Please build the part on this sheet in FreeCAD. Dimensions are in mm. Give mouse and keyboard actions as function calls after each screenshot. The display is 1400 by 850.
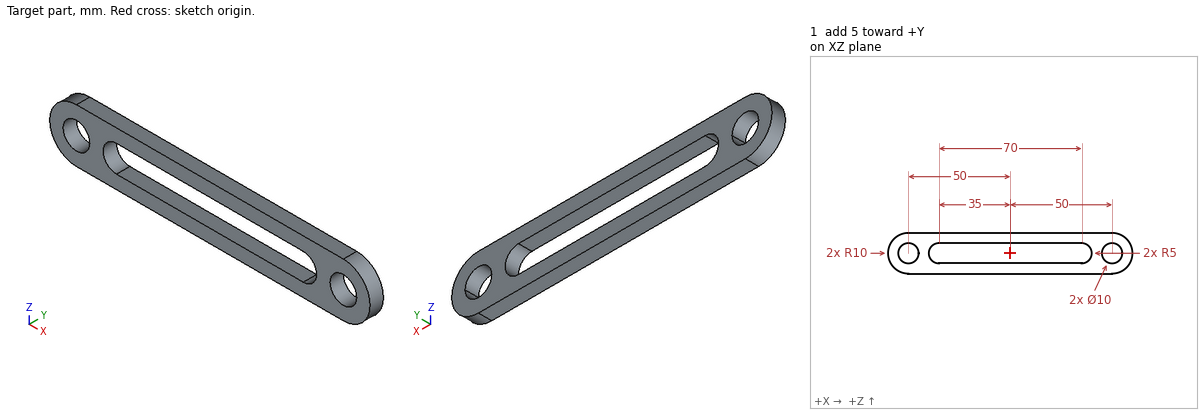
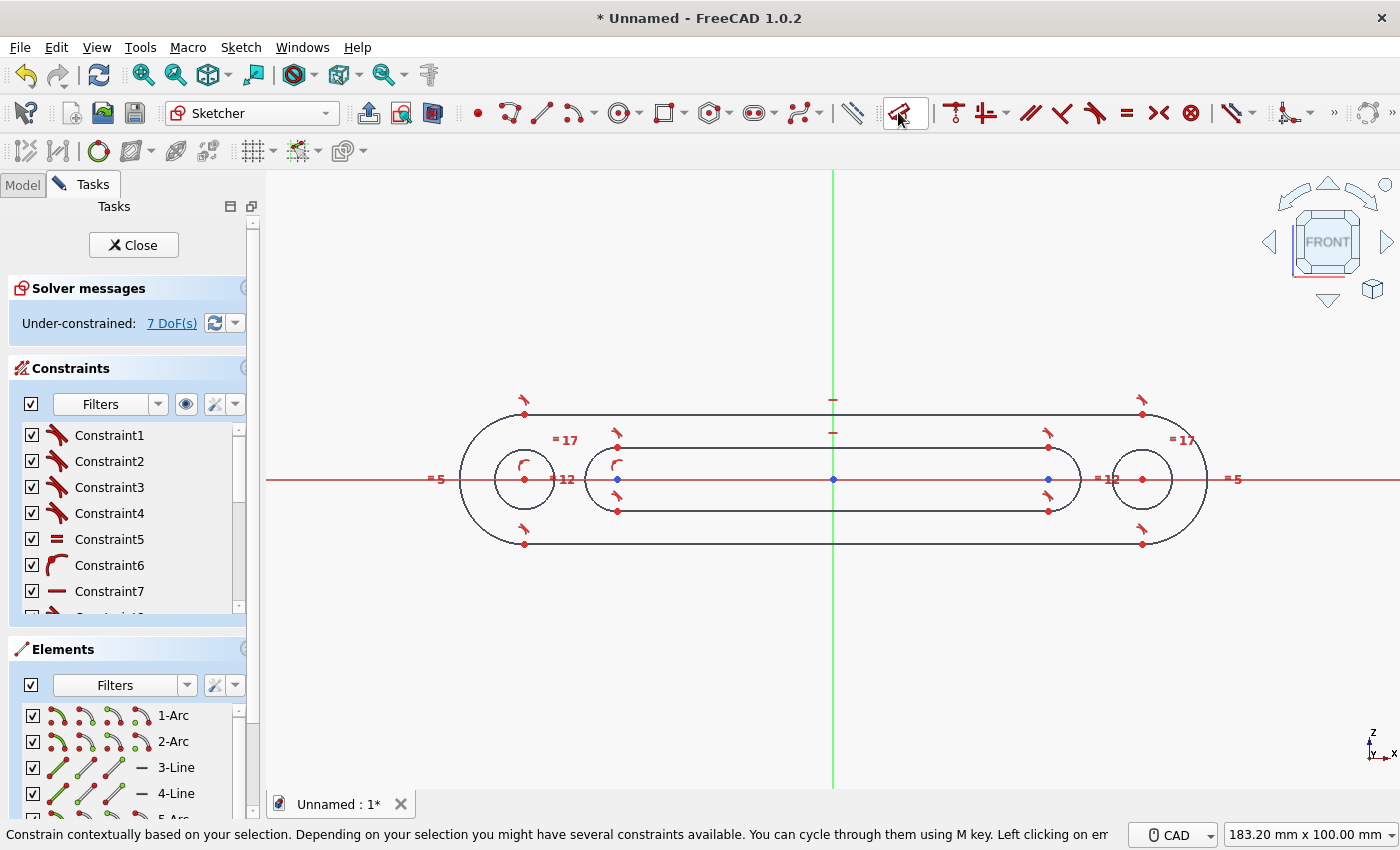
click(472, 441)
click(446, 422)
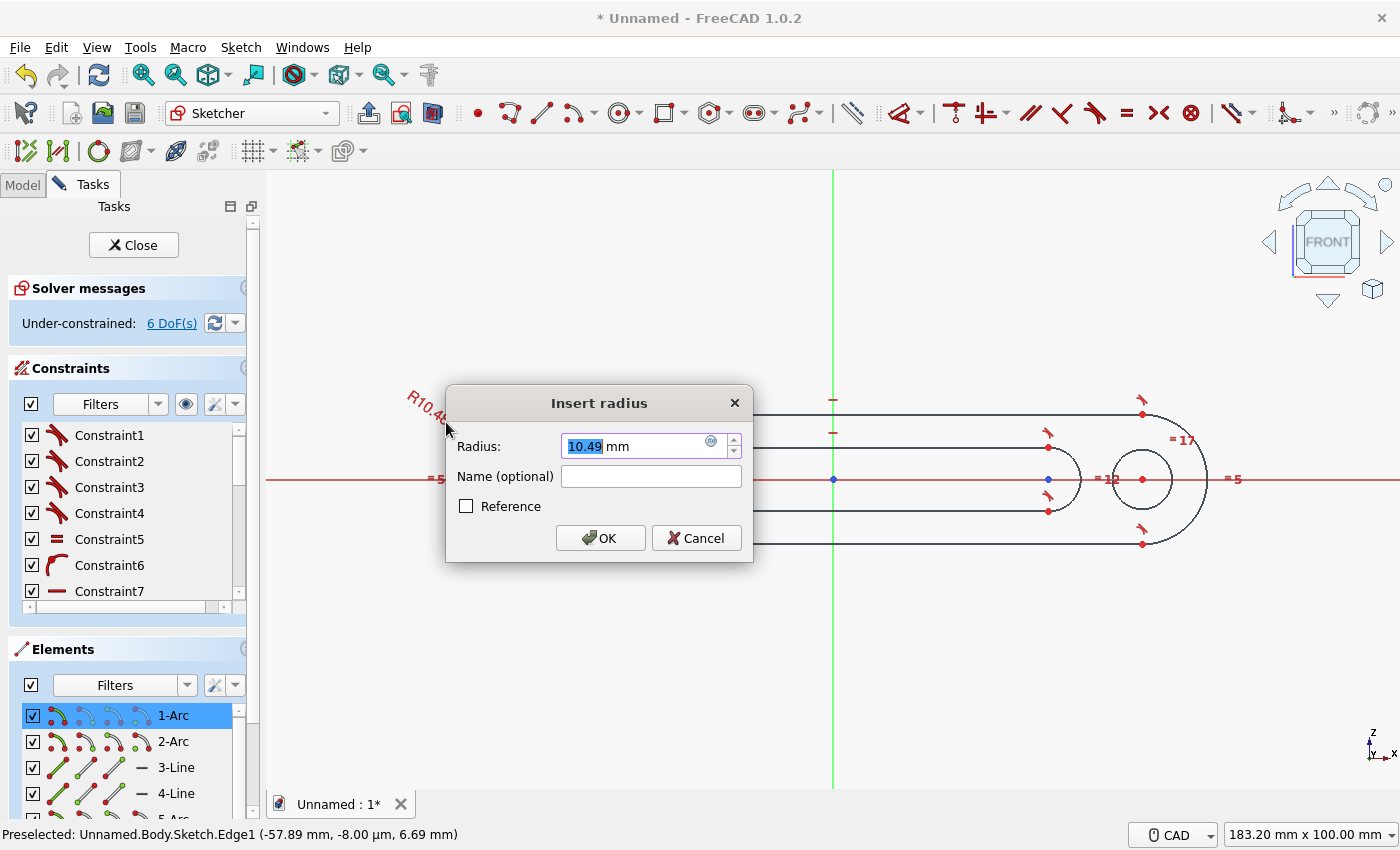
text(10)
key(Return)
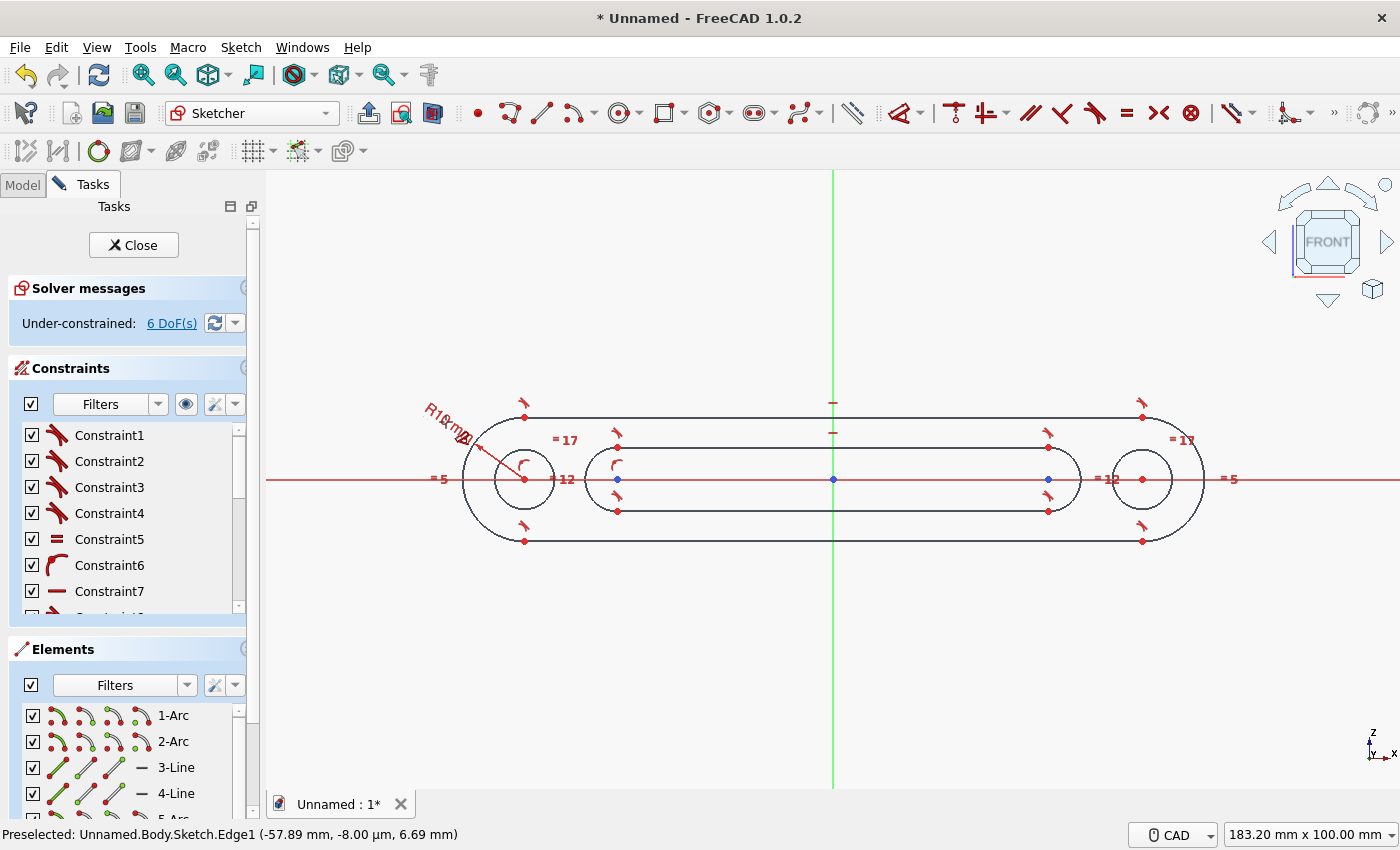
scroll(591, 461, up, 2)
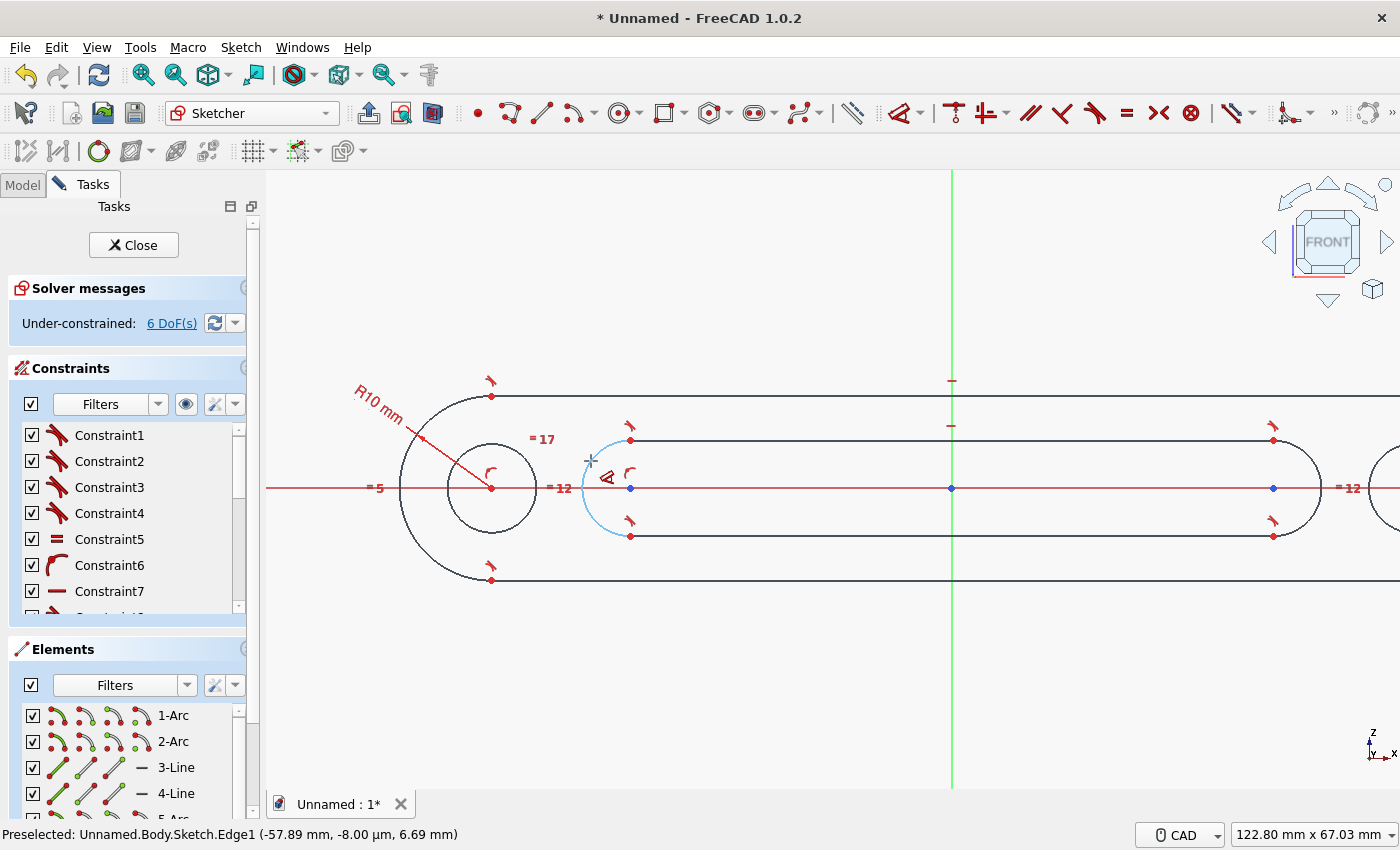
click(592, 460)
click(566, 441)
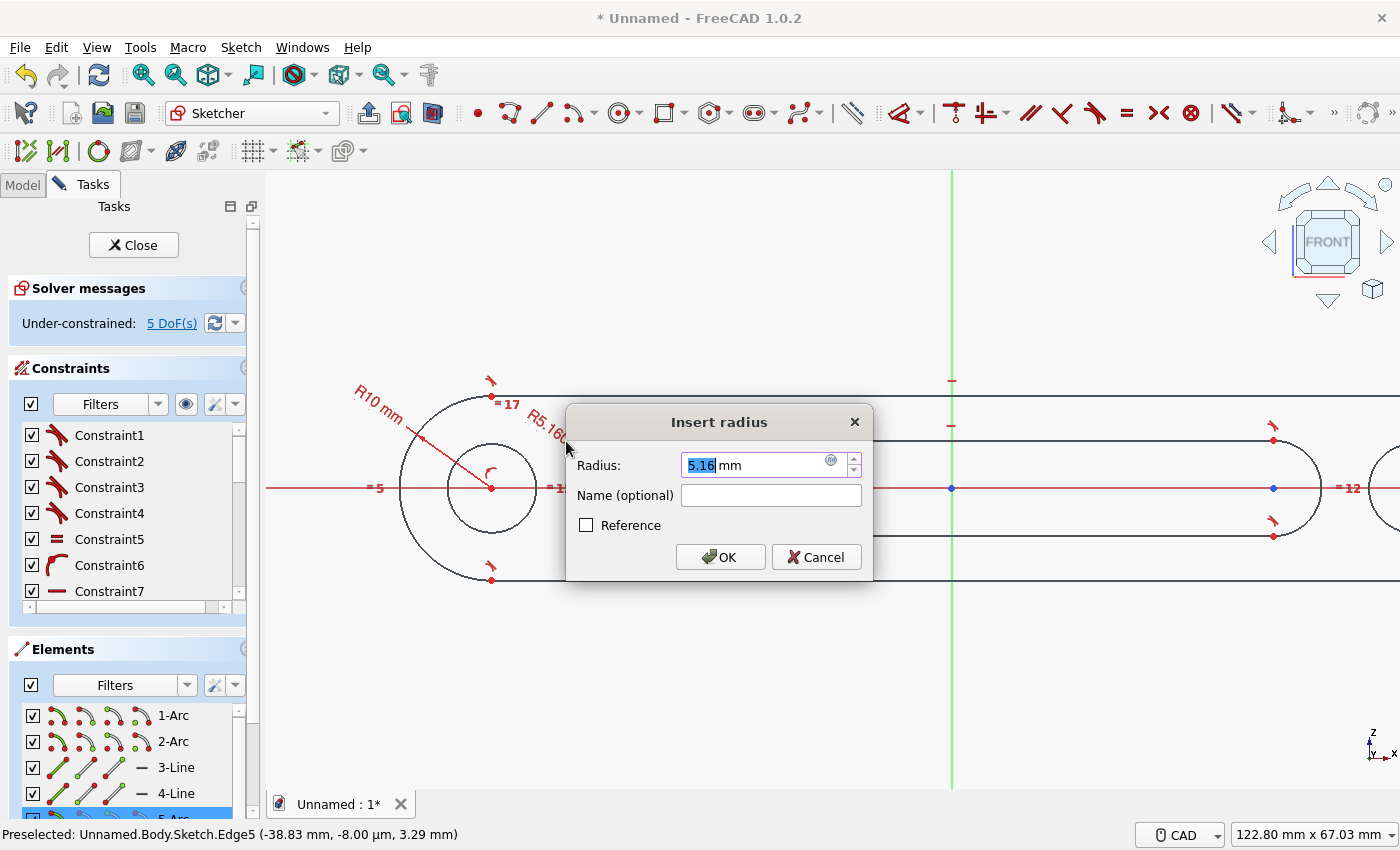
text(5)
key(Return)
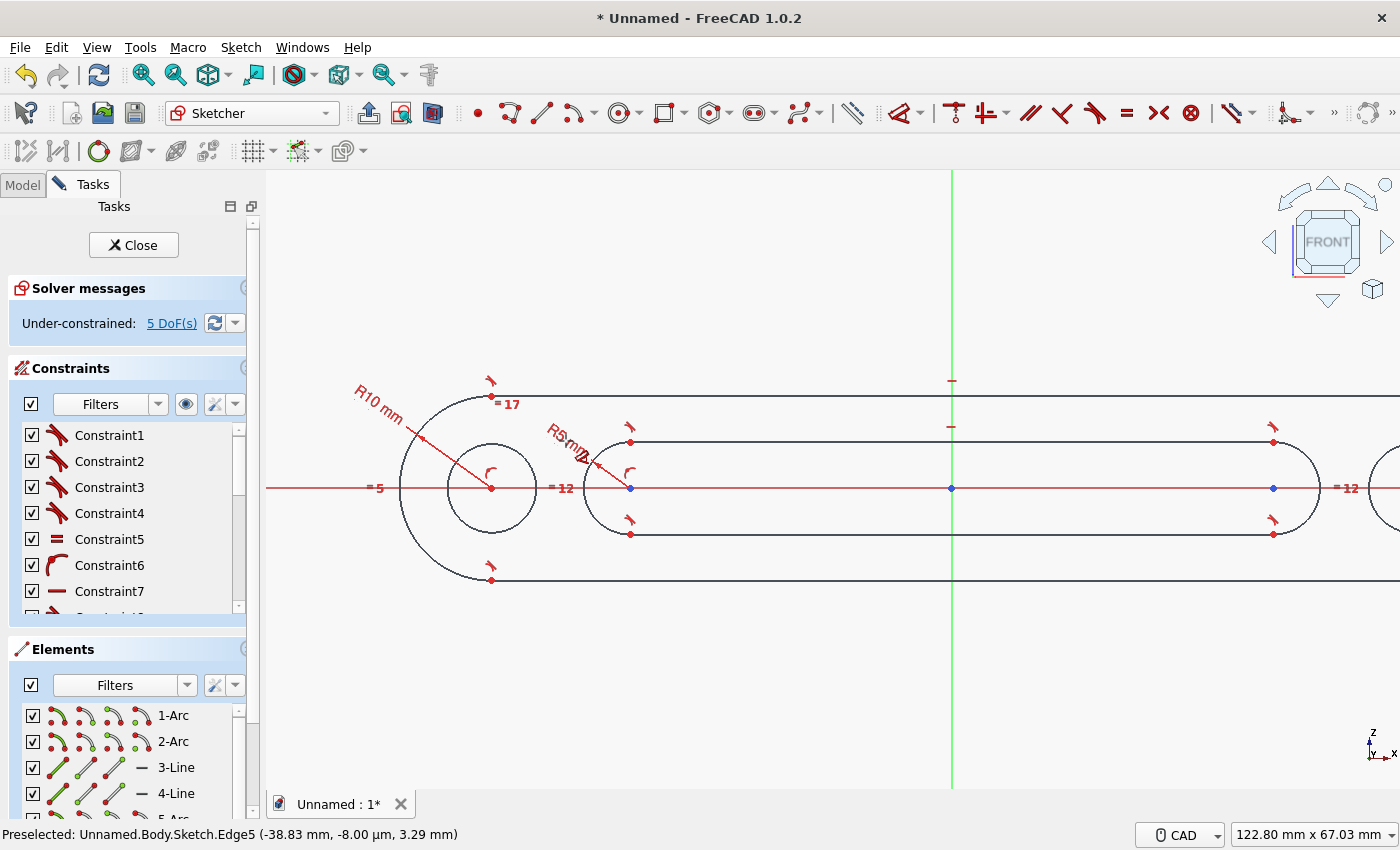
scroll(537, 469, down, 3)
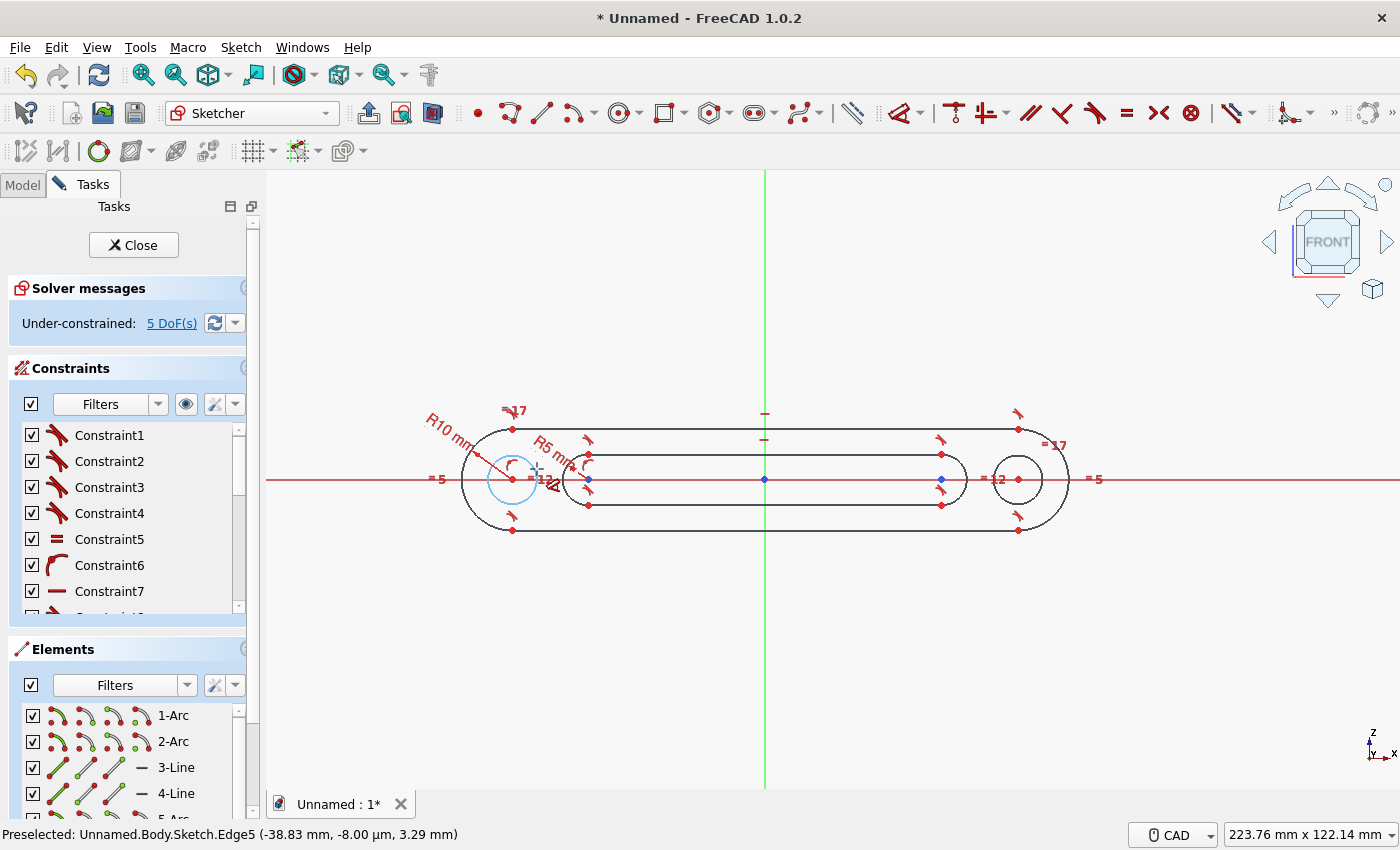
click(1035, 463)
click(1074, 424)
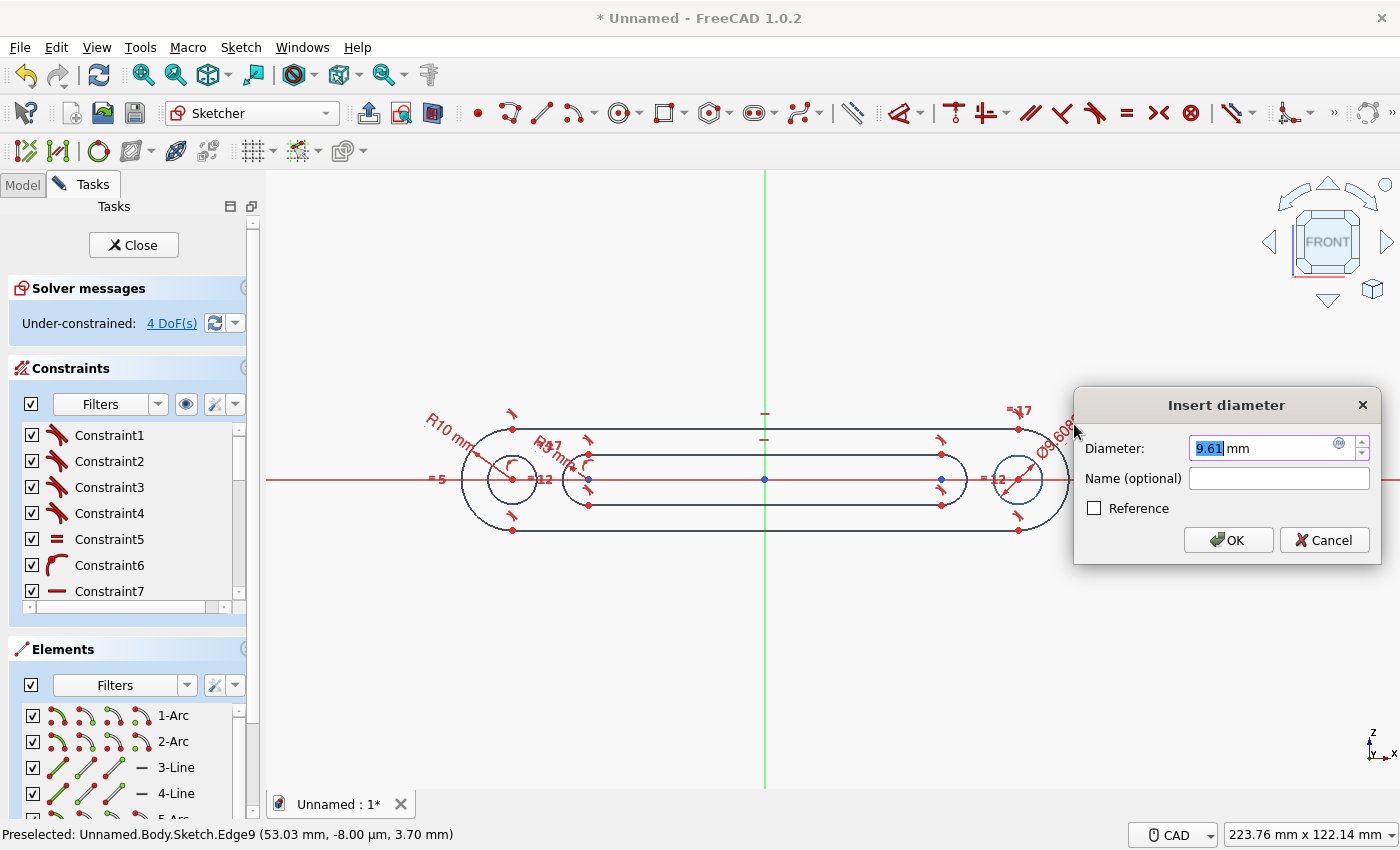
text(10)
key(Return)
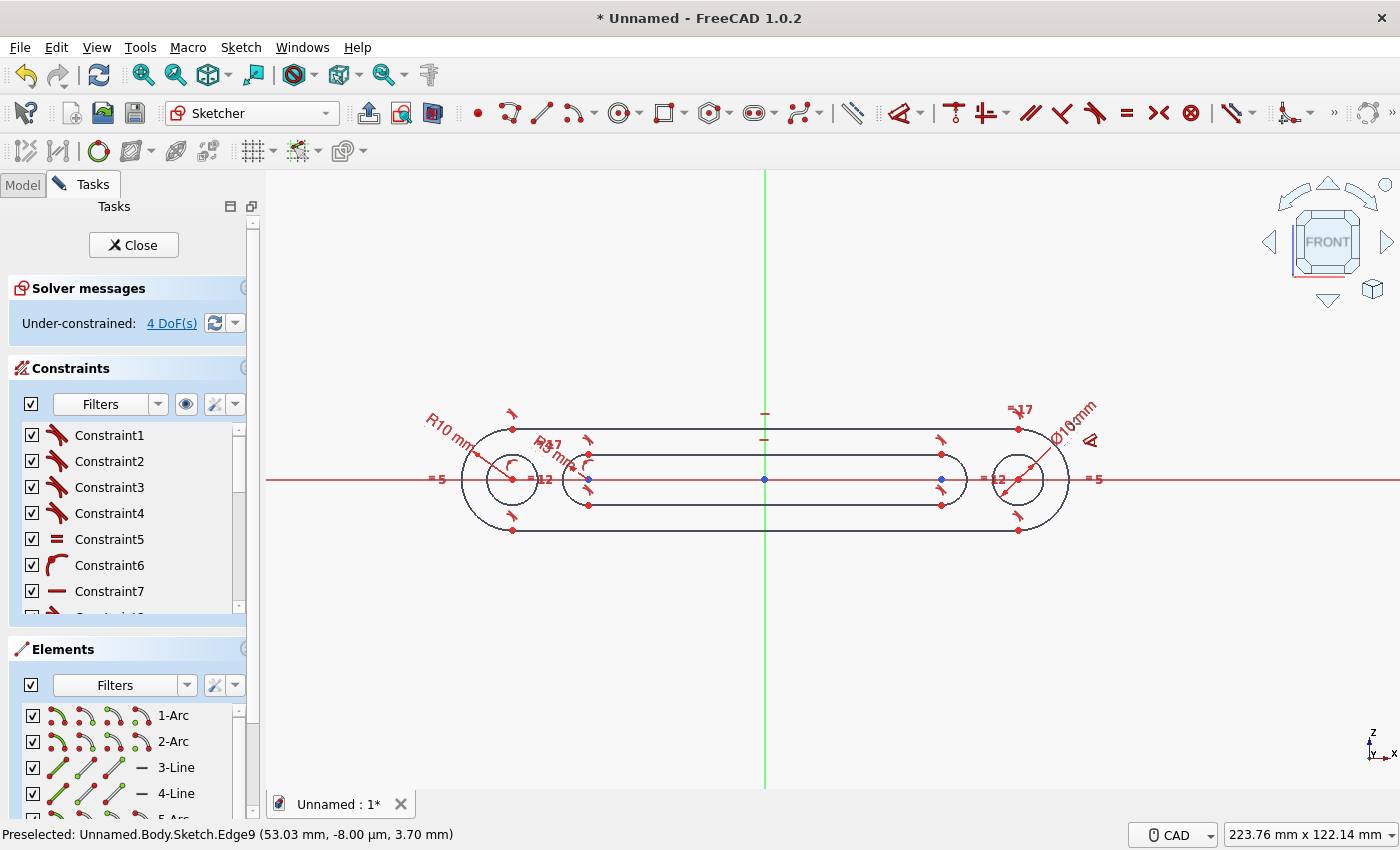
click(694, 455)
click(684, 397)